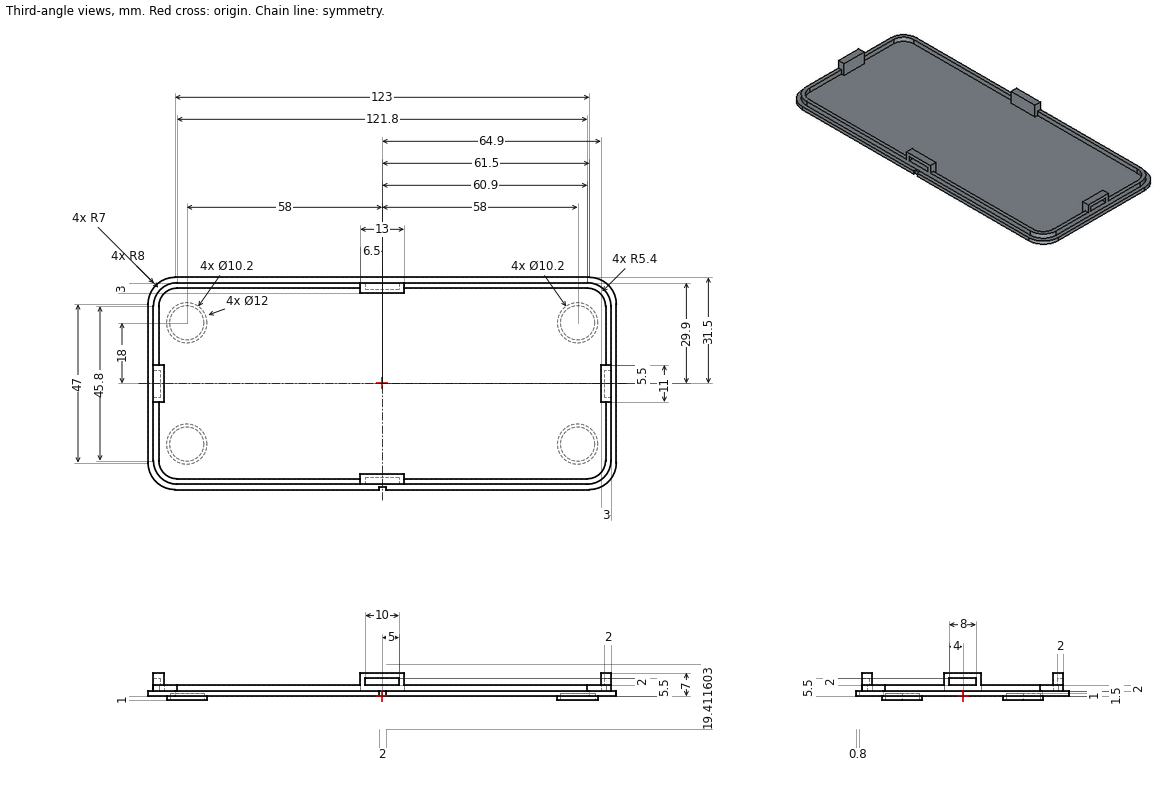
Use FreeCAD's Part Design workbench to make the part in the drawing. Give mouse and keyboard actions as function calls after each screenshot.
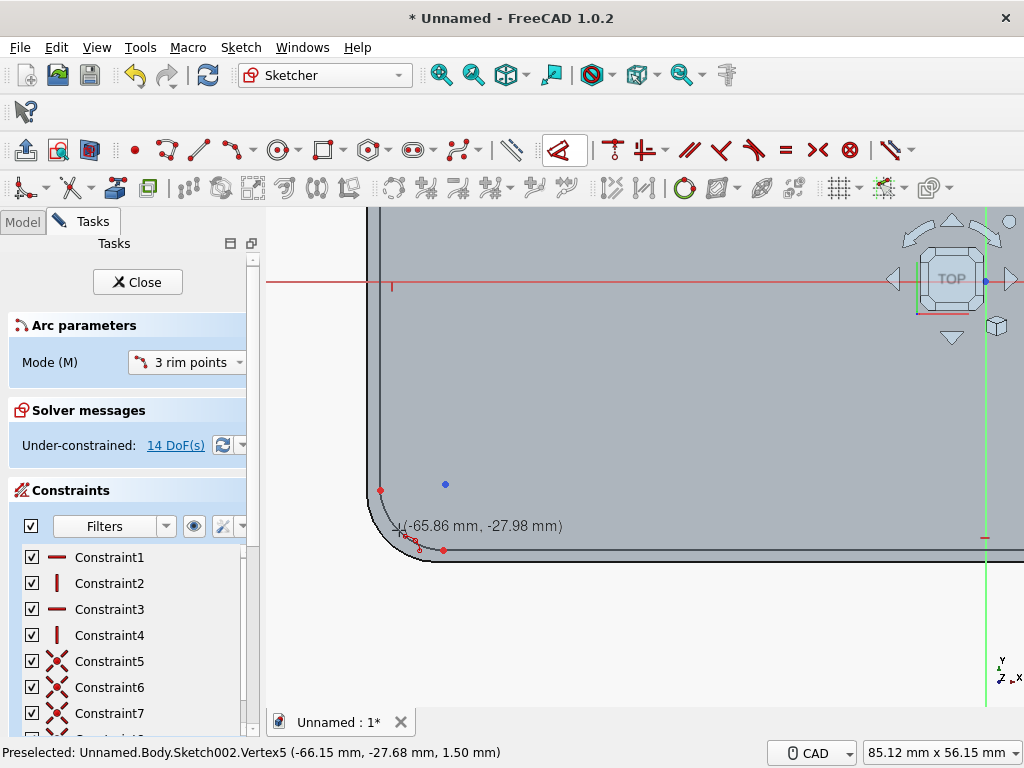
scroll(400, 533, down, 6)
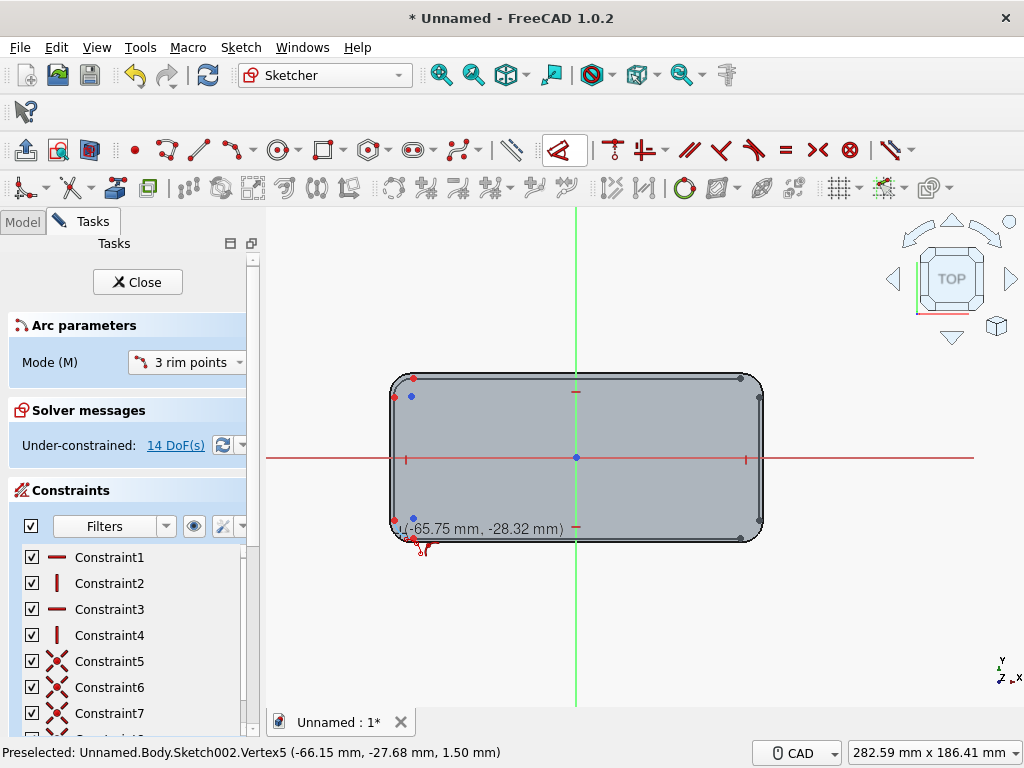
click(740, 539)
click(759, 521)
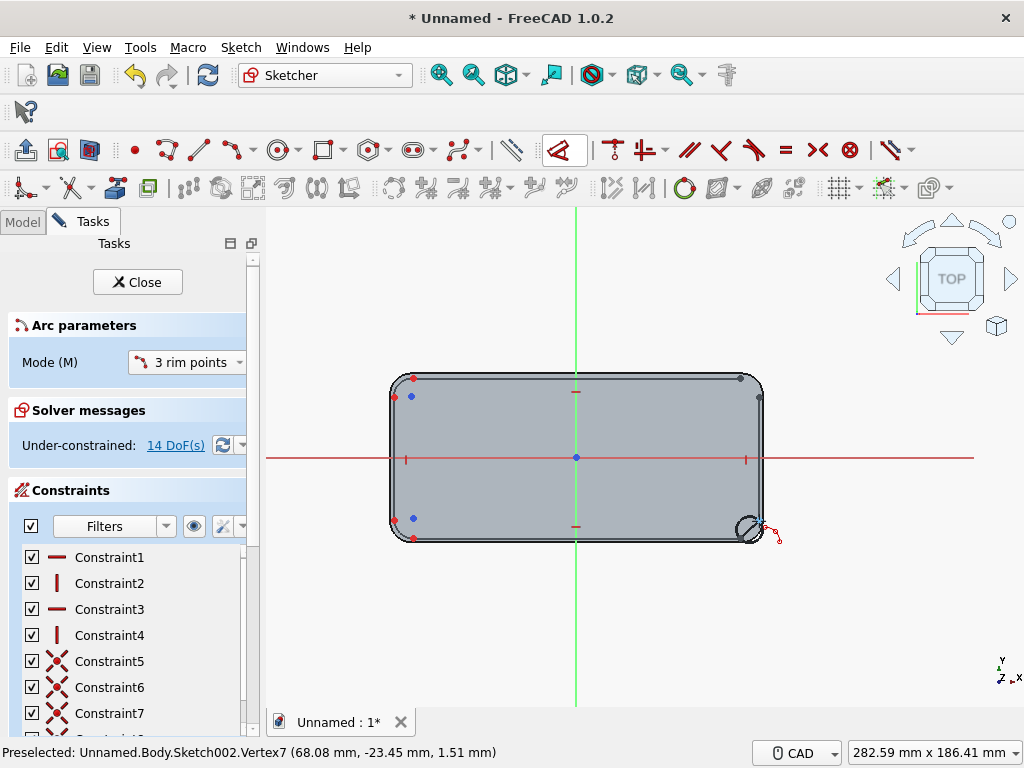
scroll(753, 532, up, 6)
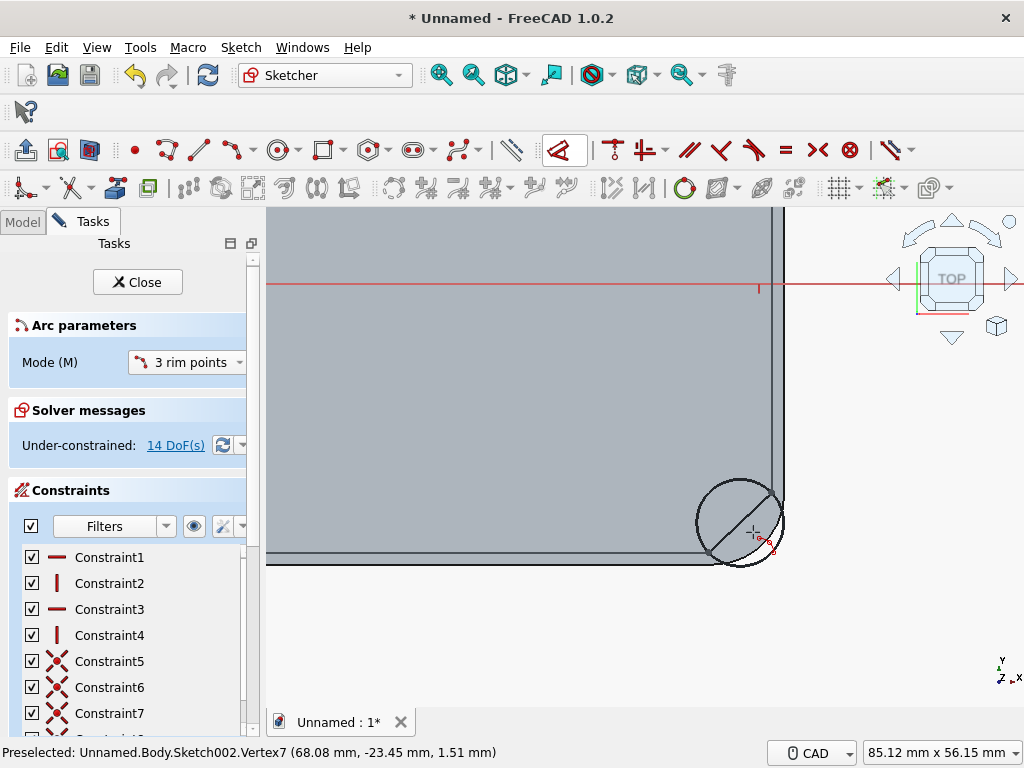
click(752, 532)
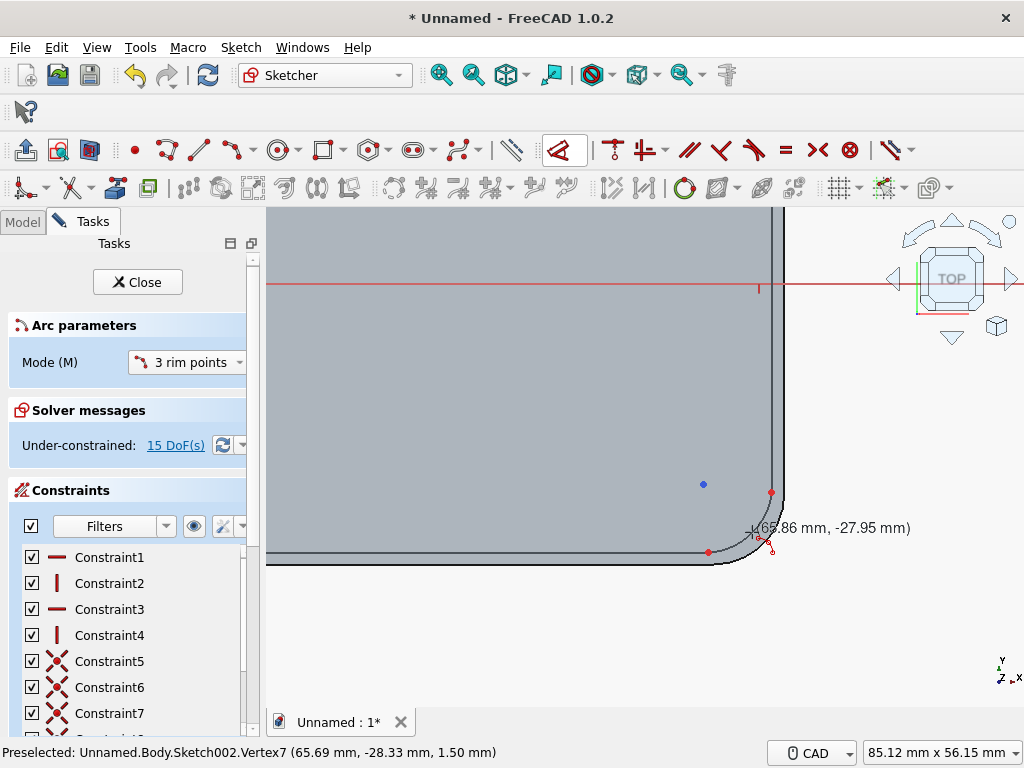
scroll(754, 532, down, 6)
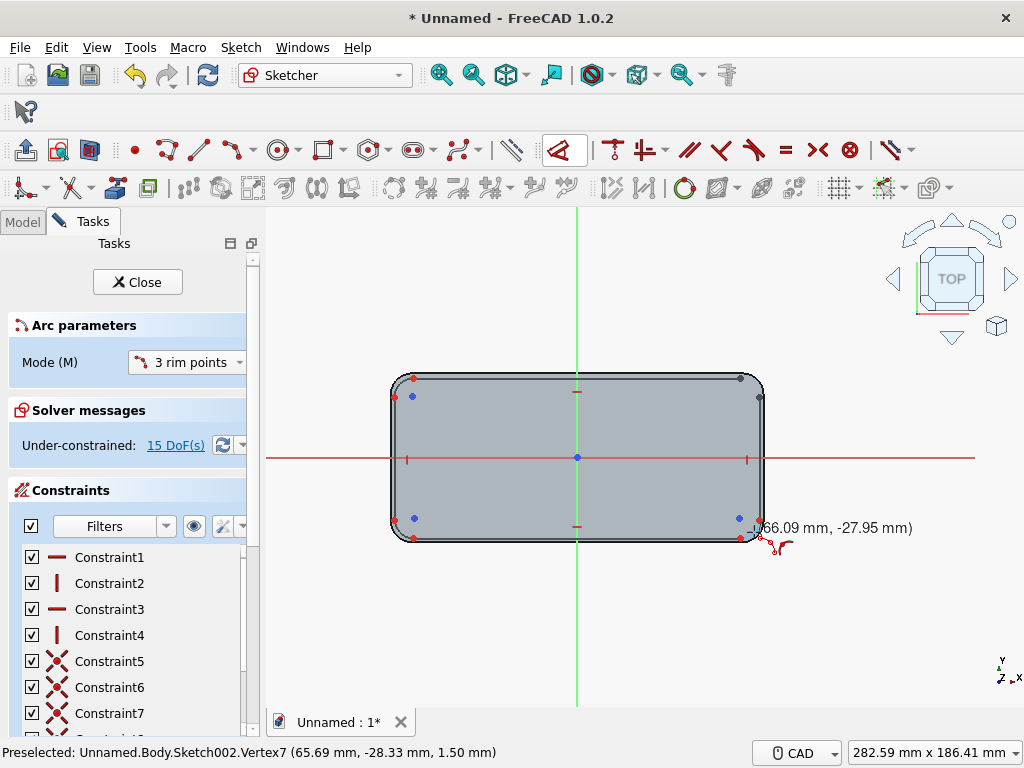
click(760, 398)
click(741, 379)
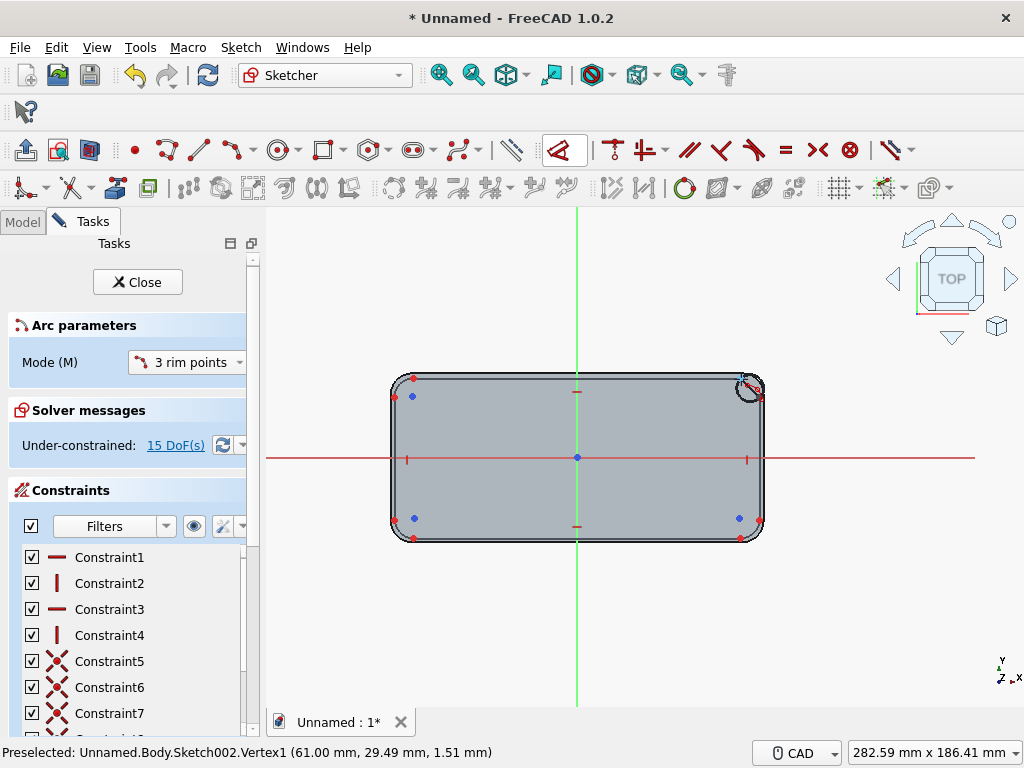
scroll(754, 383, up, 6)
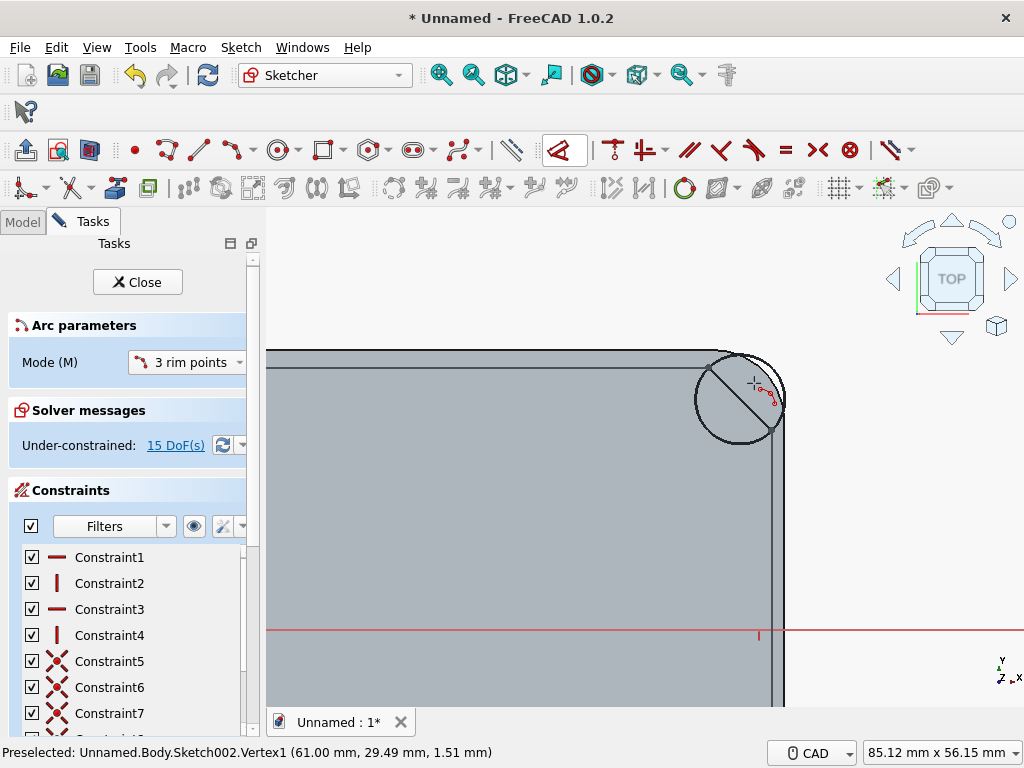
click(752, 382)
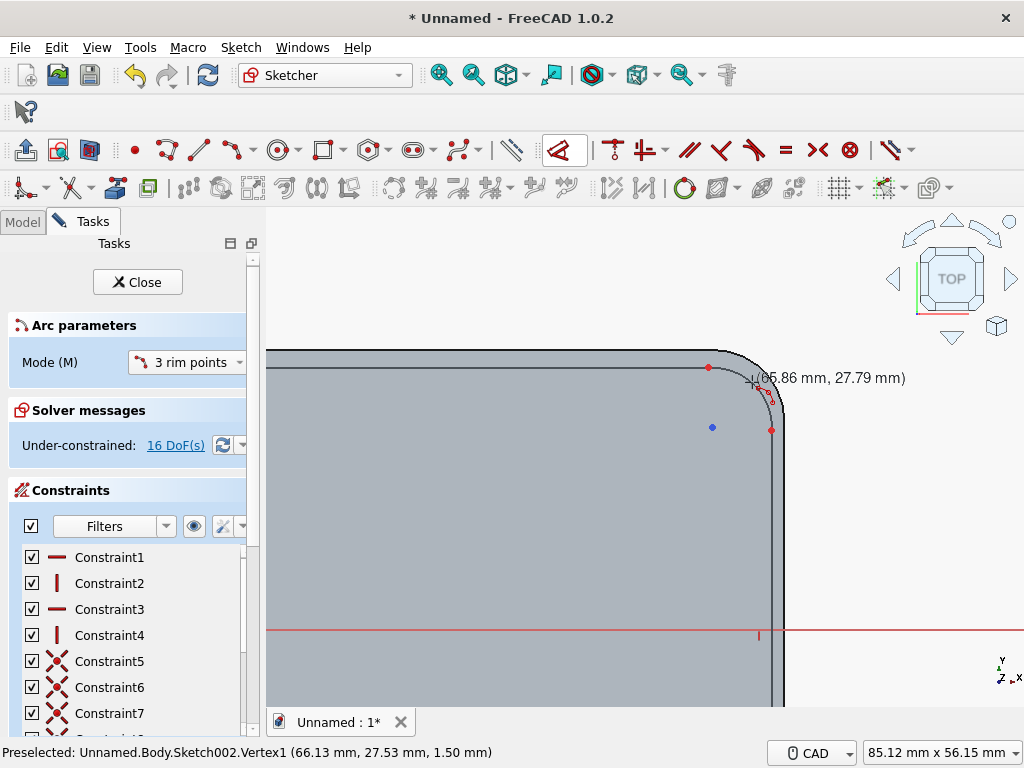
key(g)
key(l)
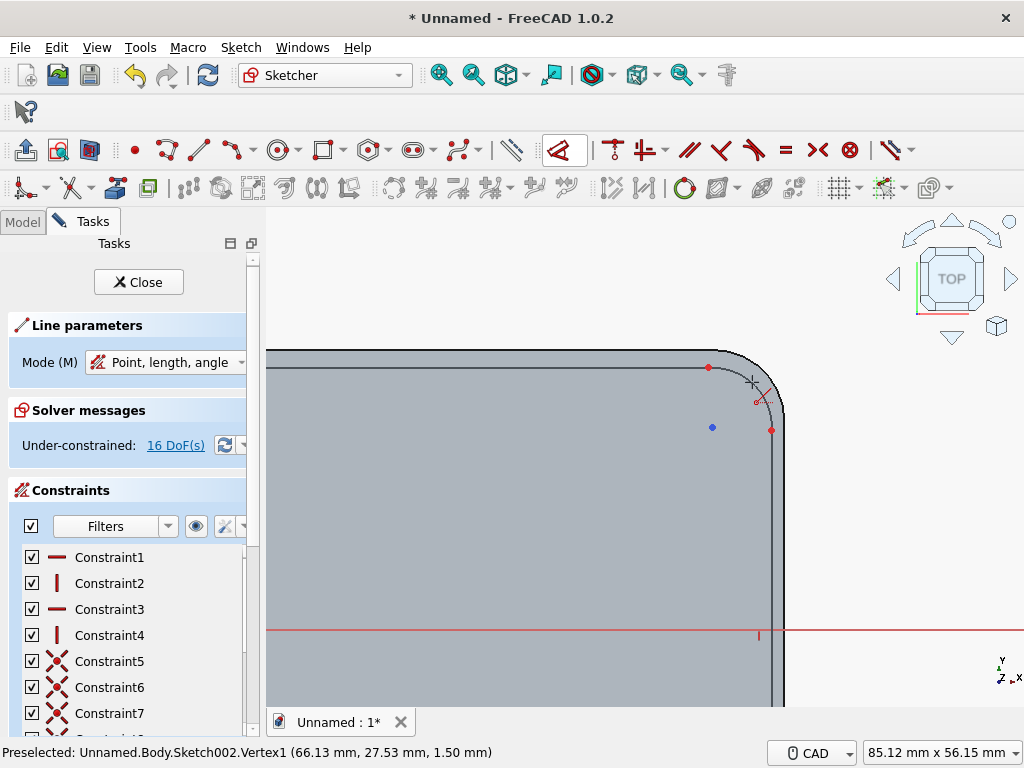
scroll(754, 382, down, 6)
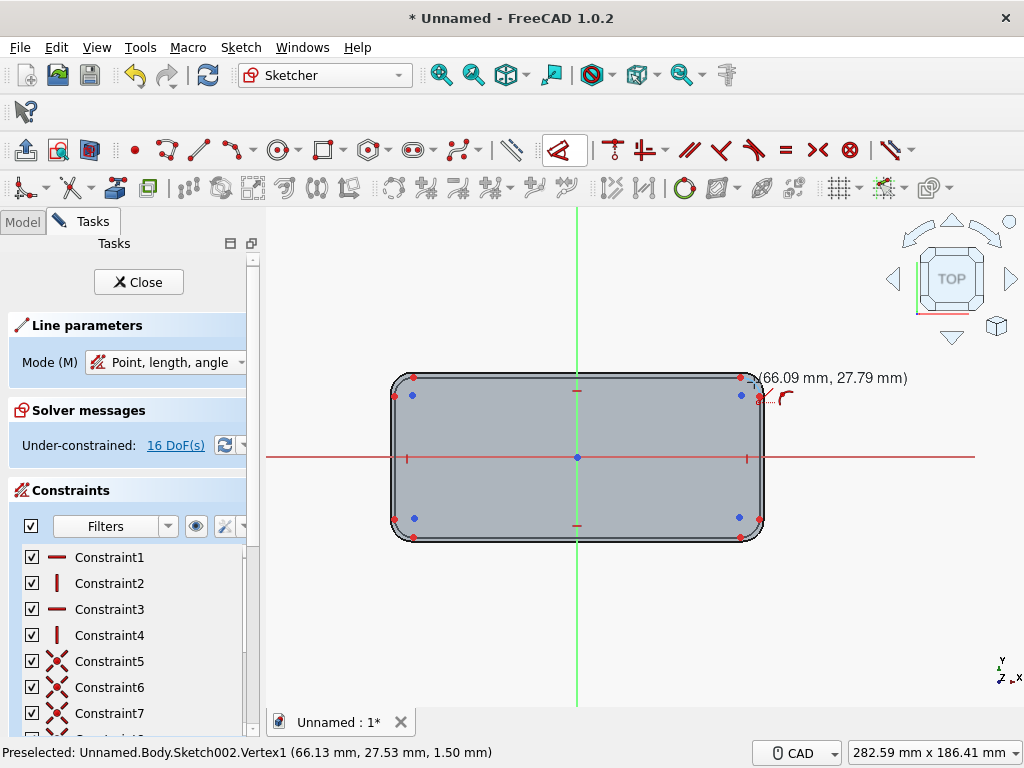
scroll(414, 381, up, 7)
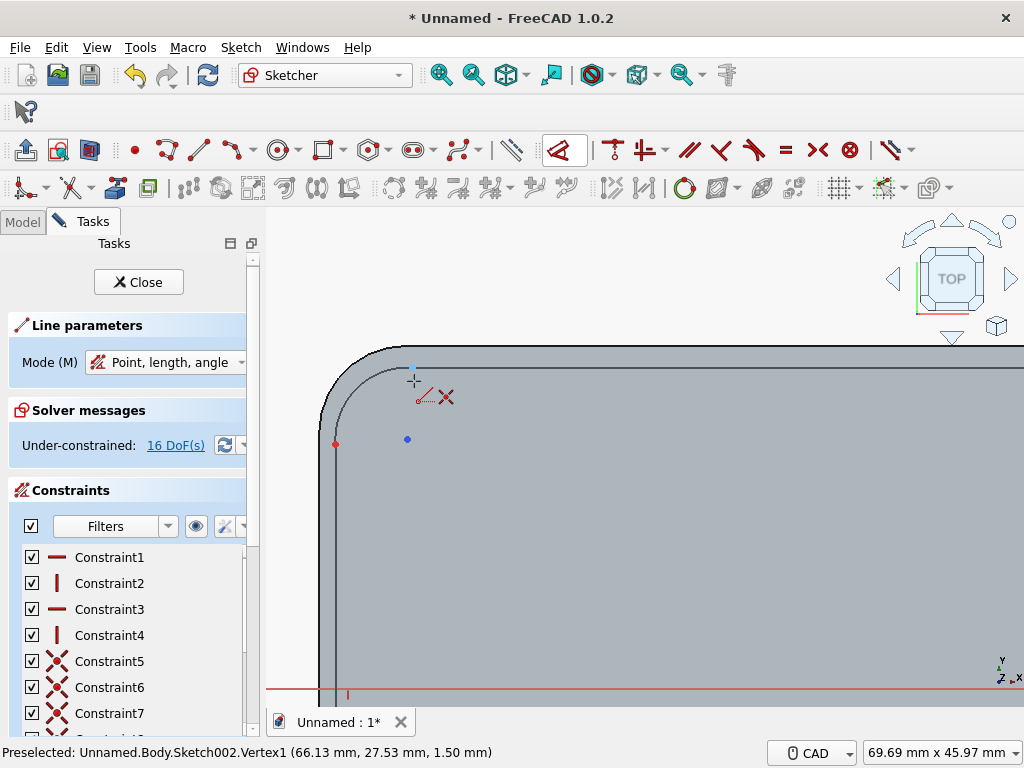
click(413, 381)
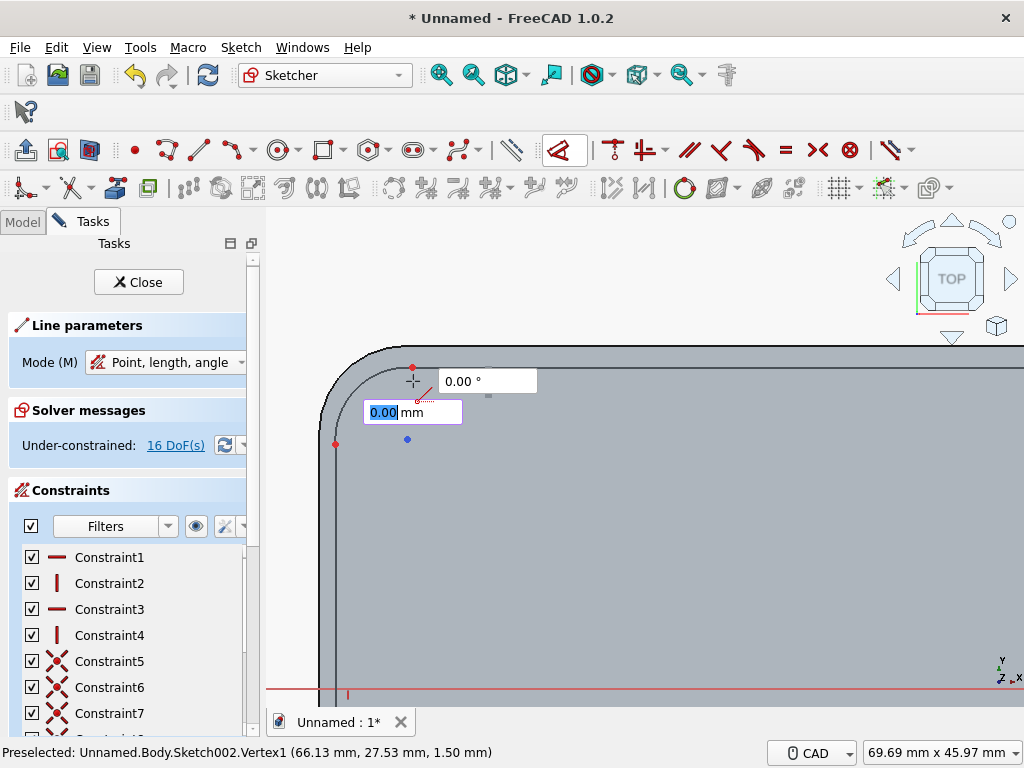
scroll(413, 381, down, 7)